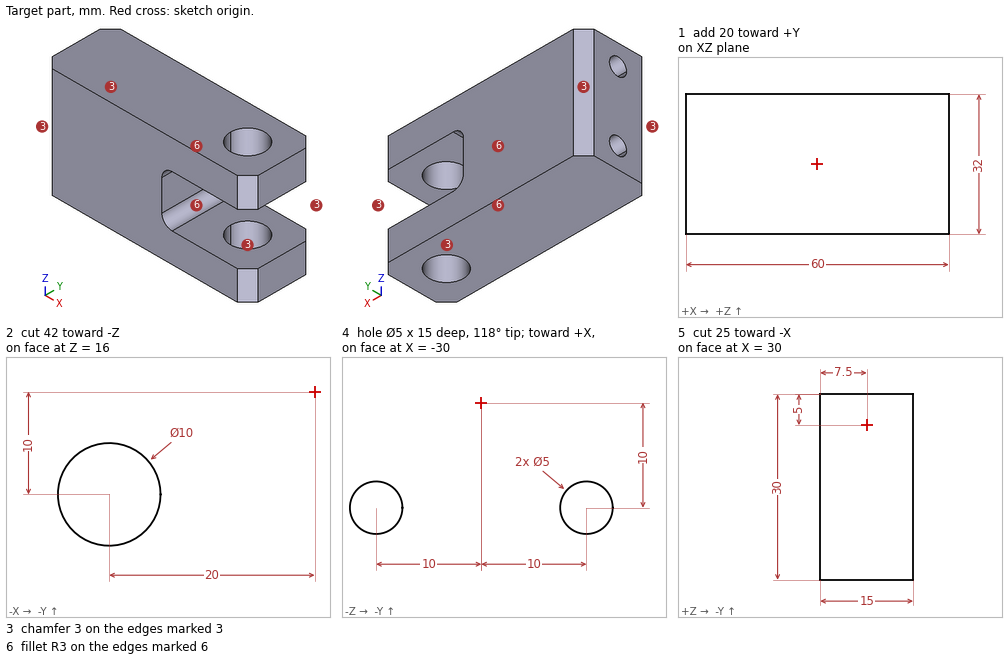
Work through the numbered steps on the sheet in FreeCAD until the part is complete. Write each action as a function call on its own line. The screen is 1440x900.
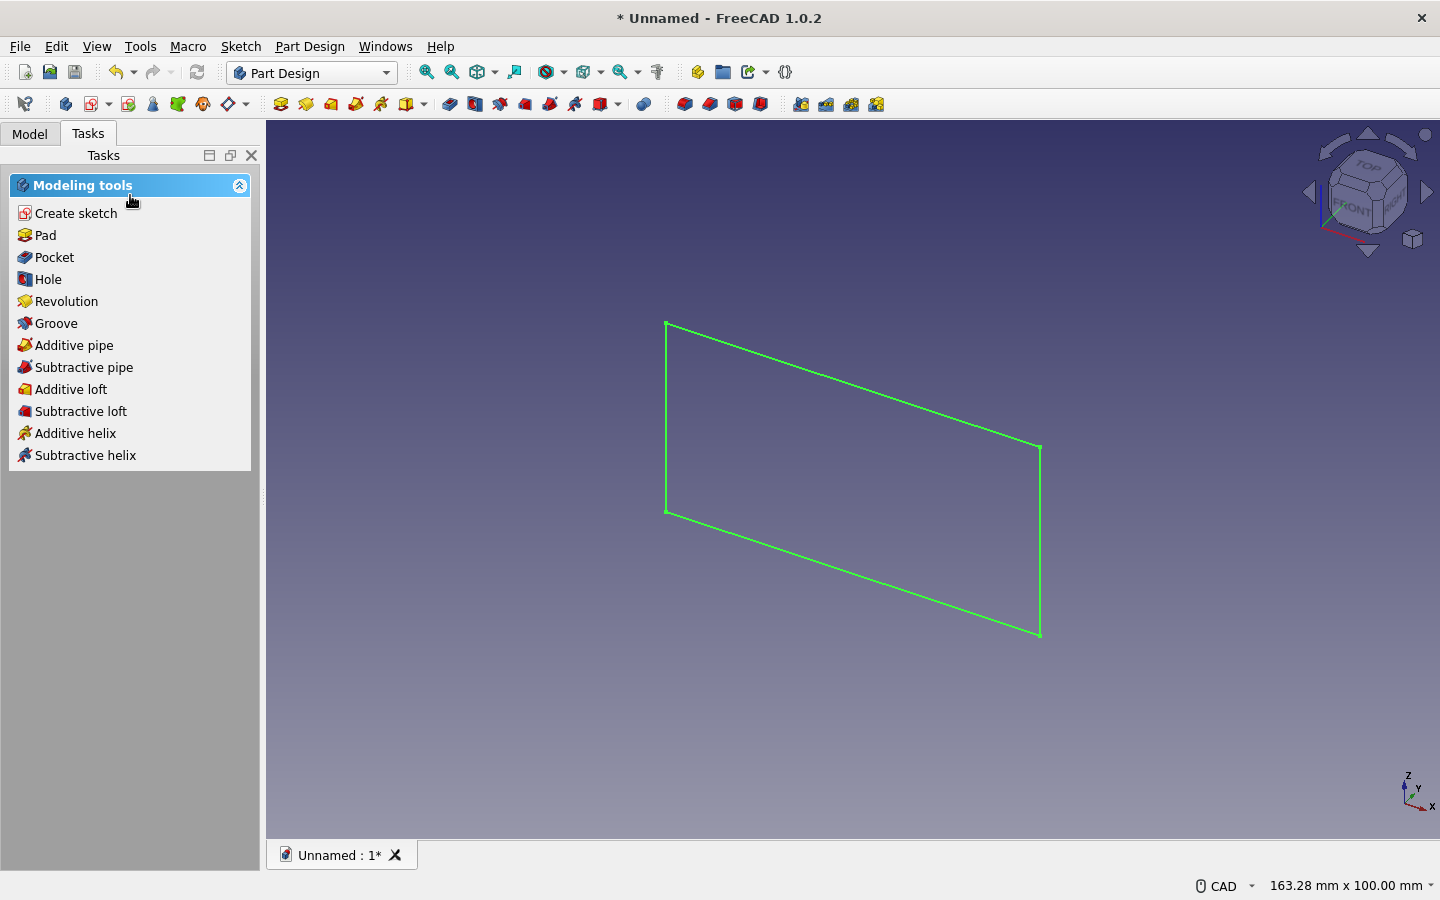
click(281, 104)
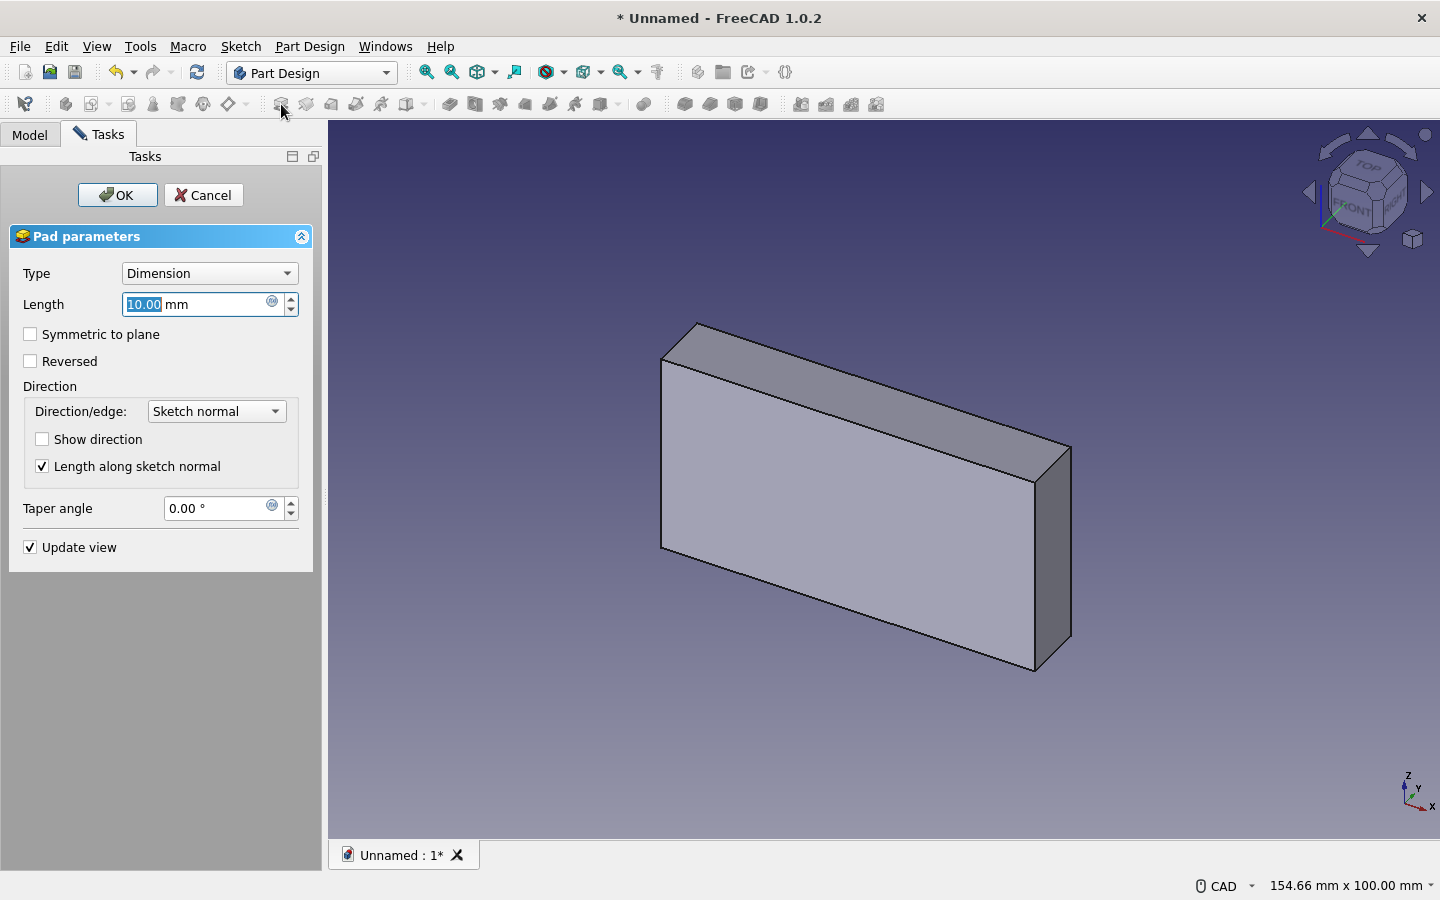
text(20)
key(Tab)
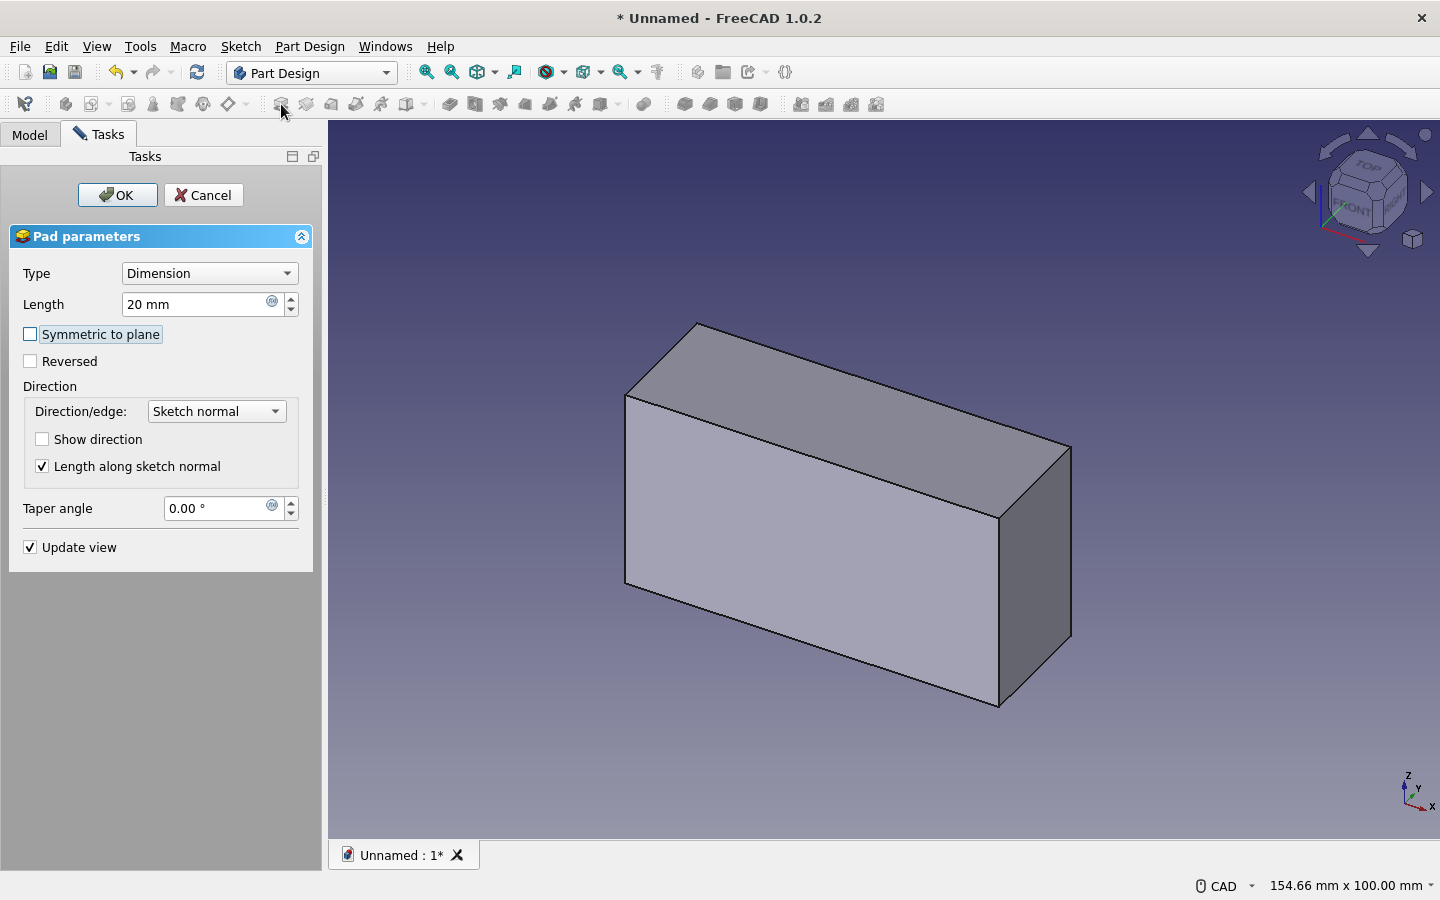
click(31, 361)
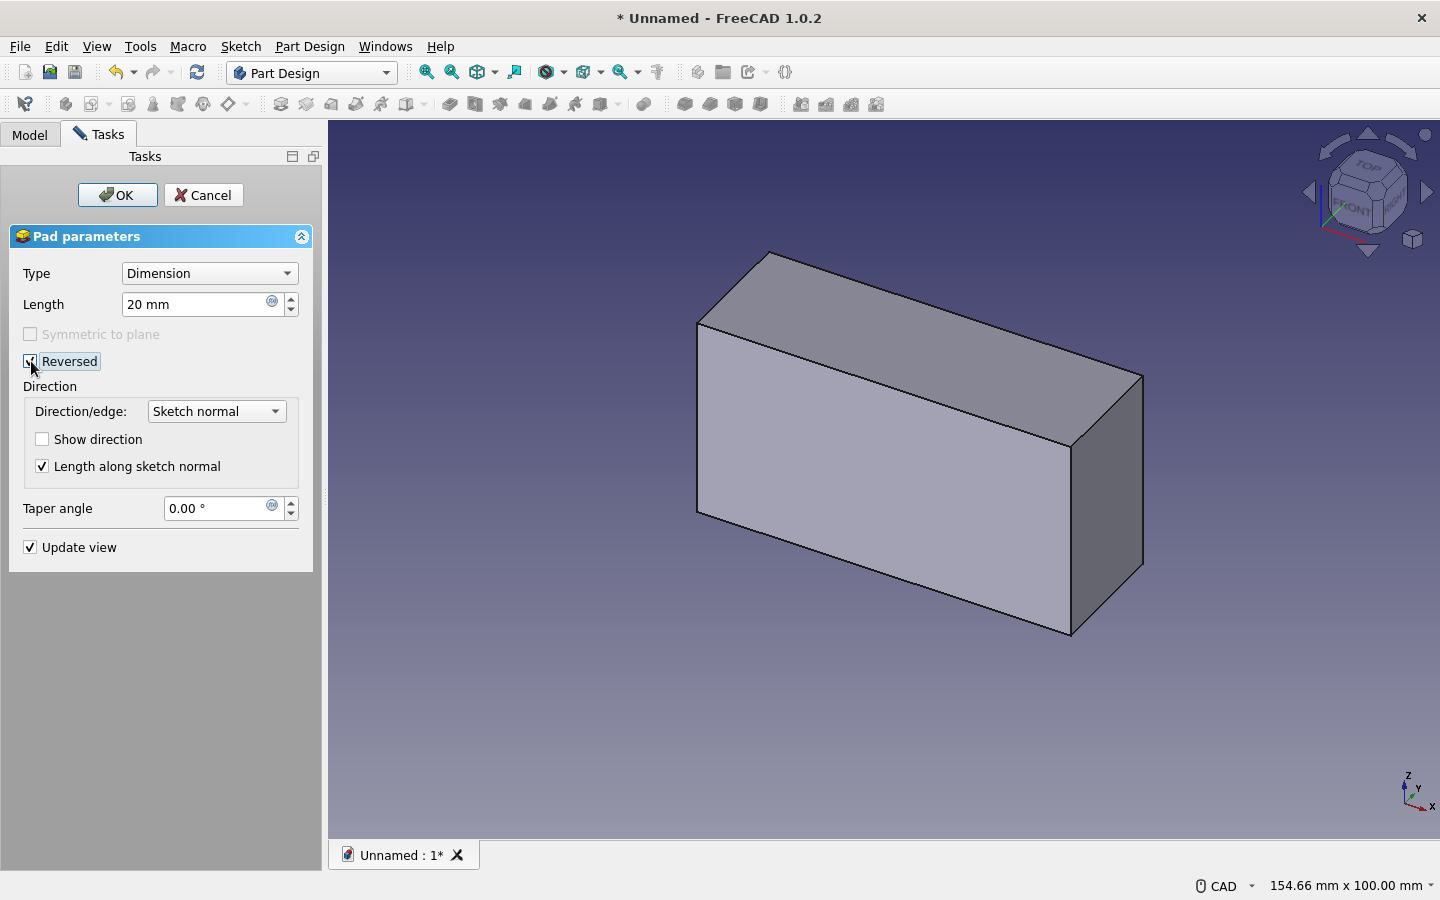
click(118, 195)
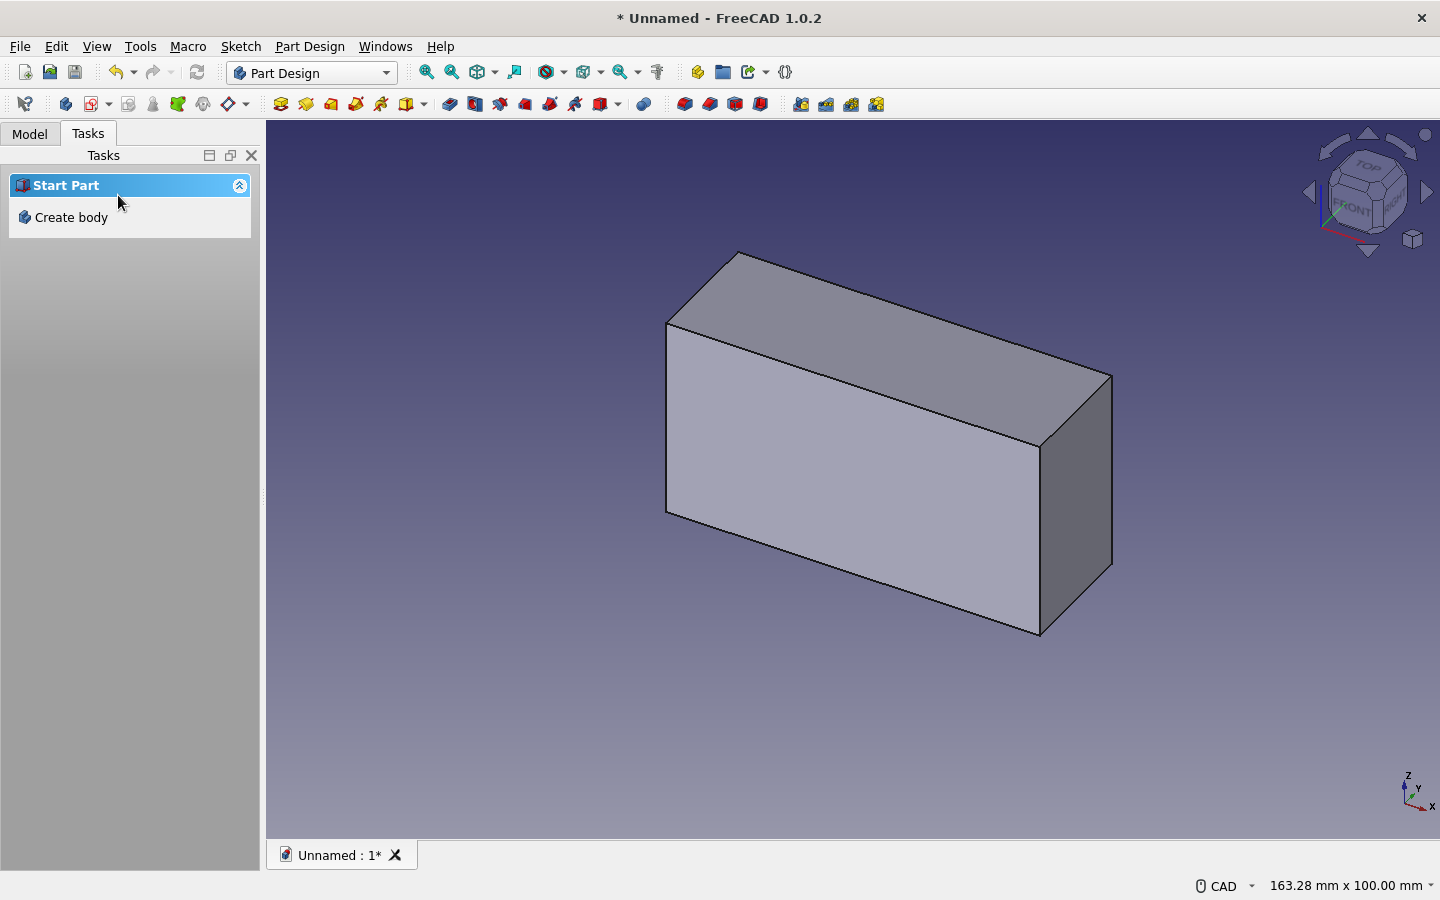
click(996, 384)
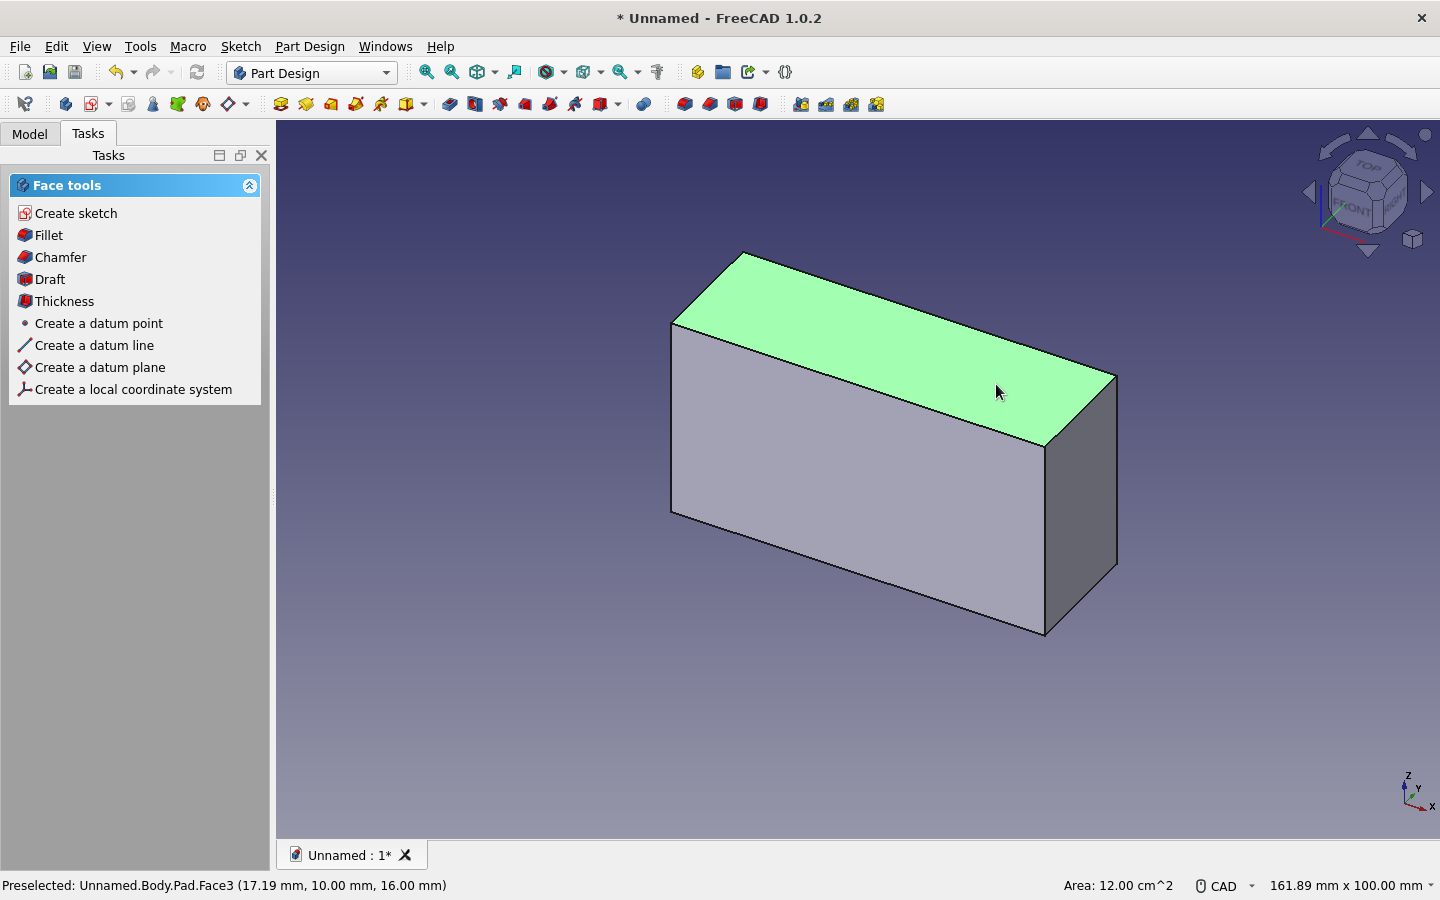
click(90, 104)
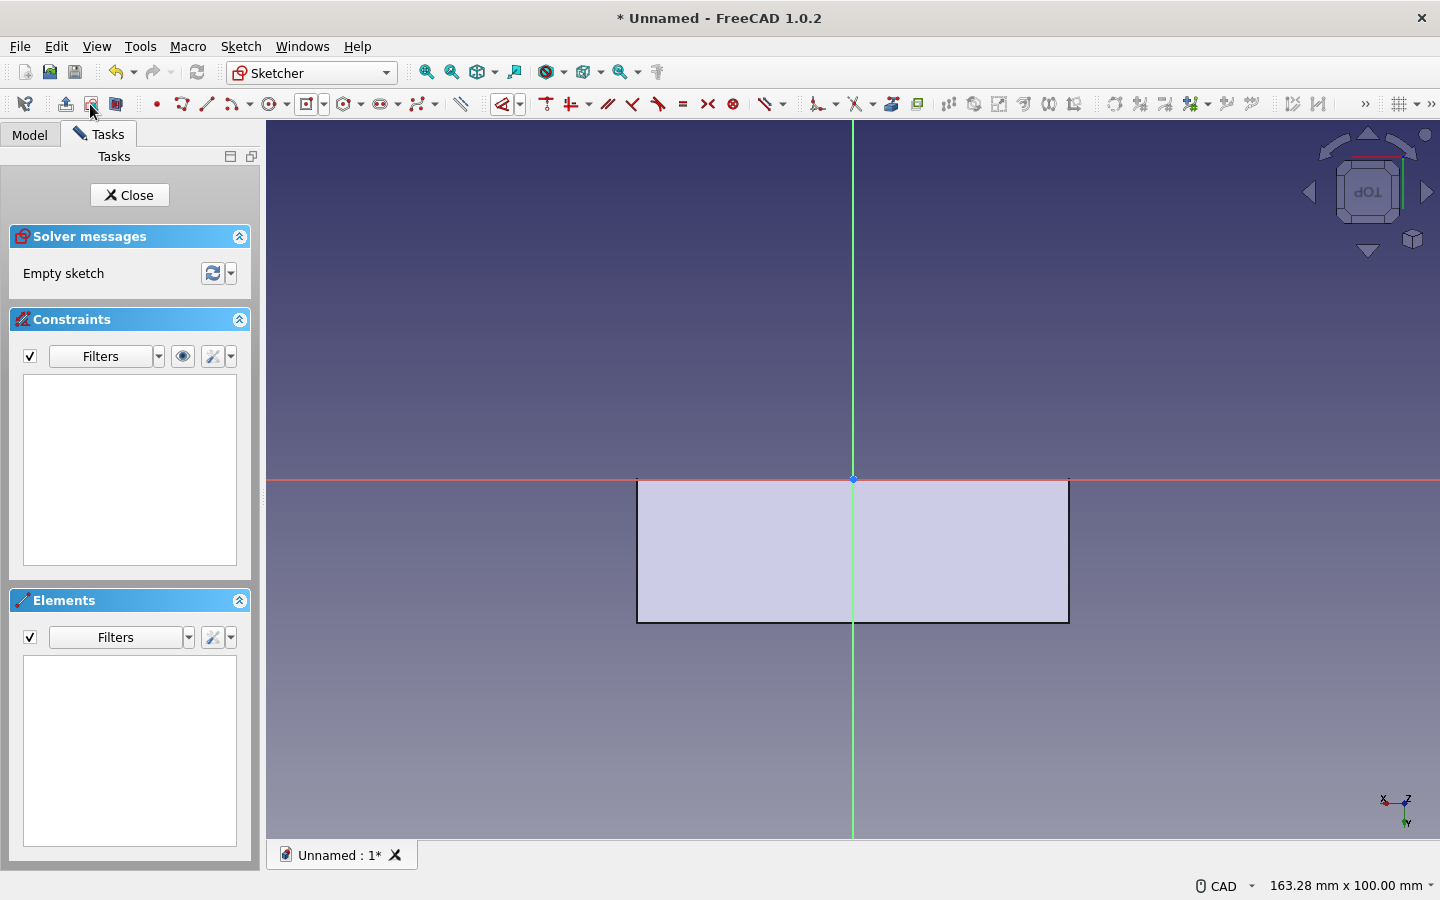
scroll(694, 566, up, 9)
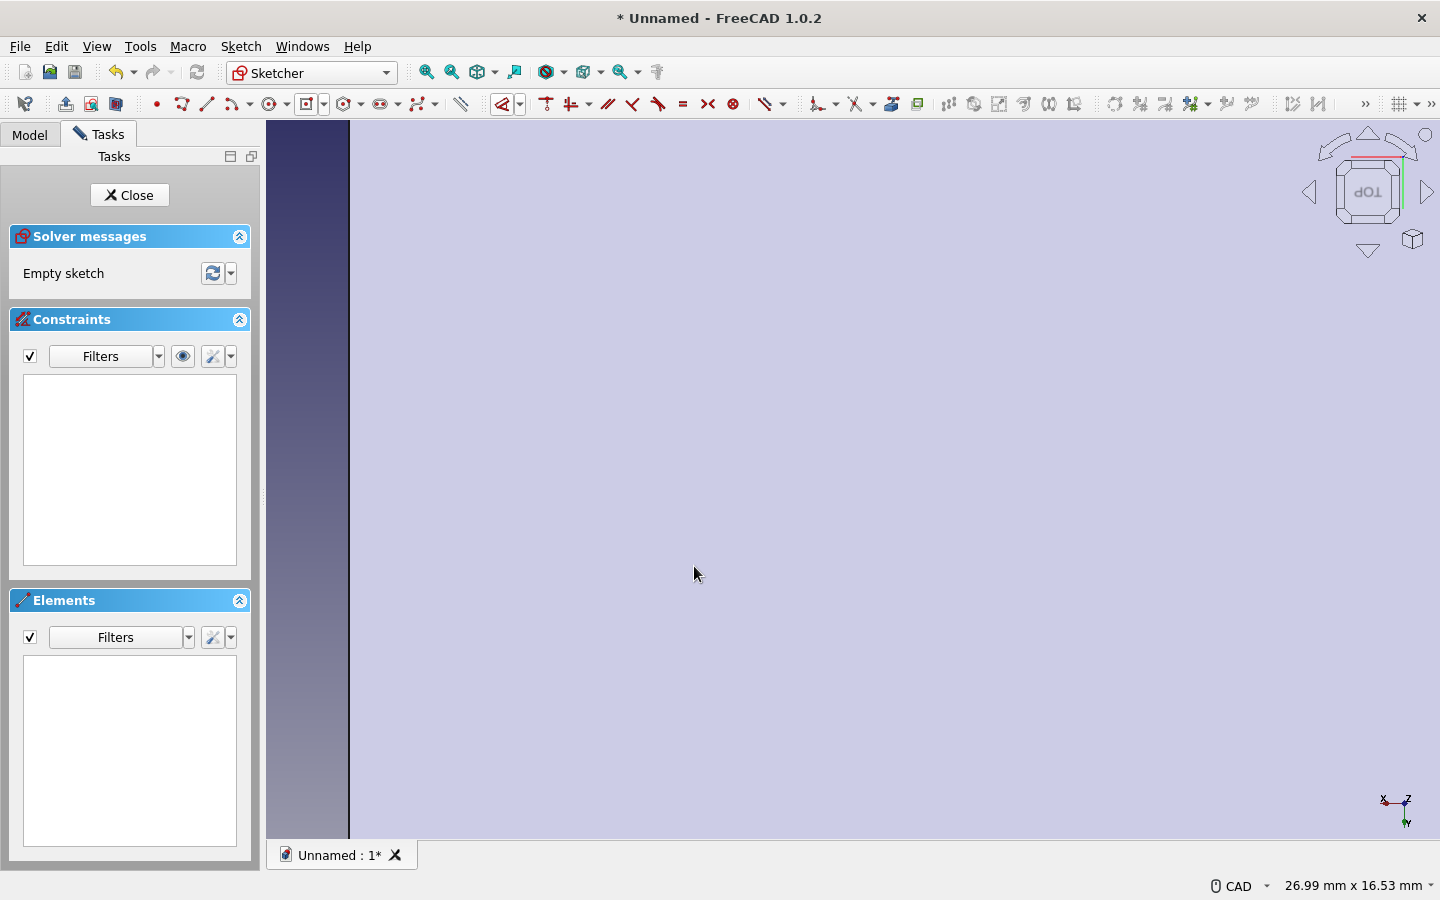
click(268, 104)